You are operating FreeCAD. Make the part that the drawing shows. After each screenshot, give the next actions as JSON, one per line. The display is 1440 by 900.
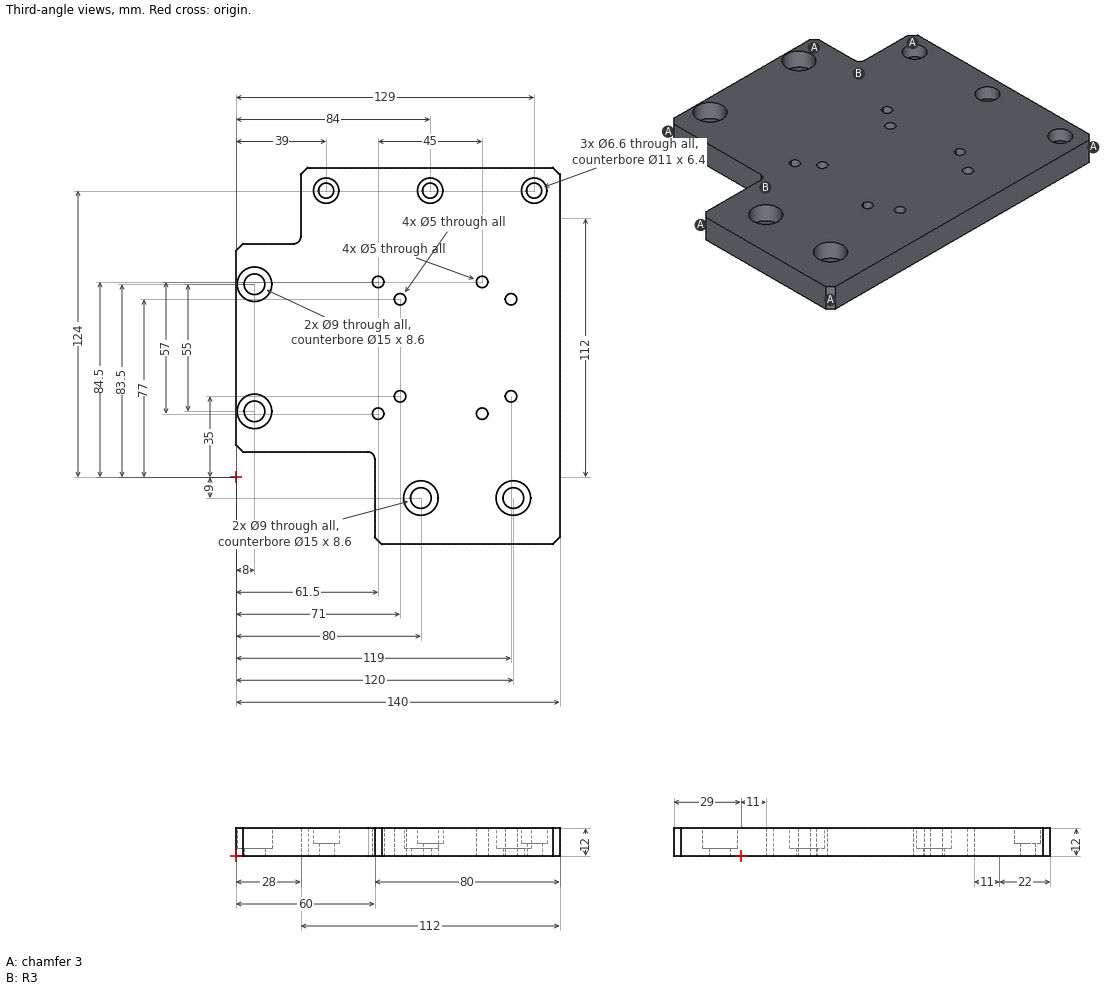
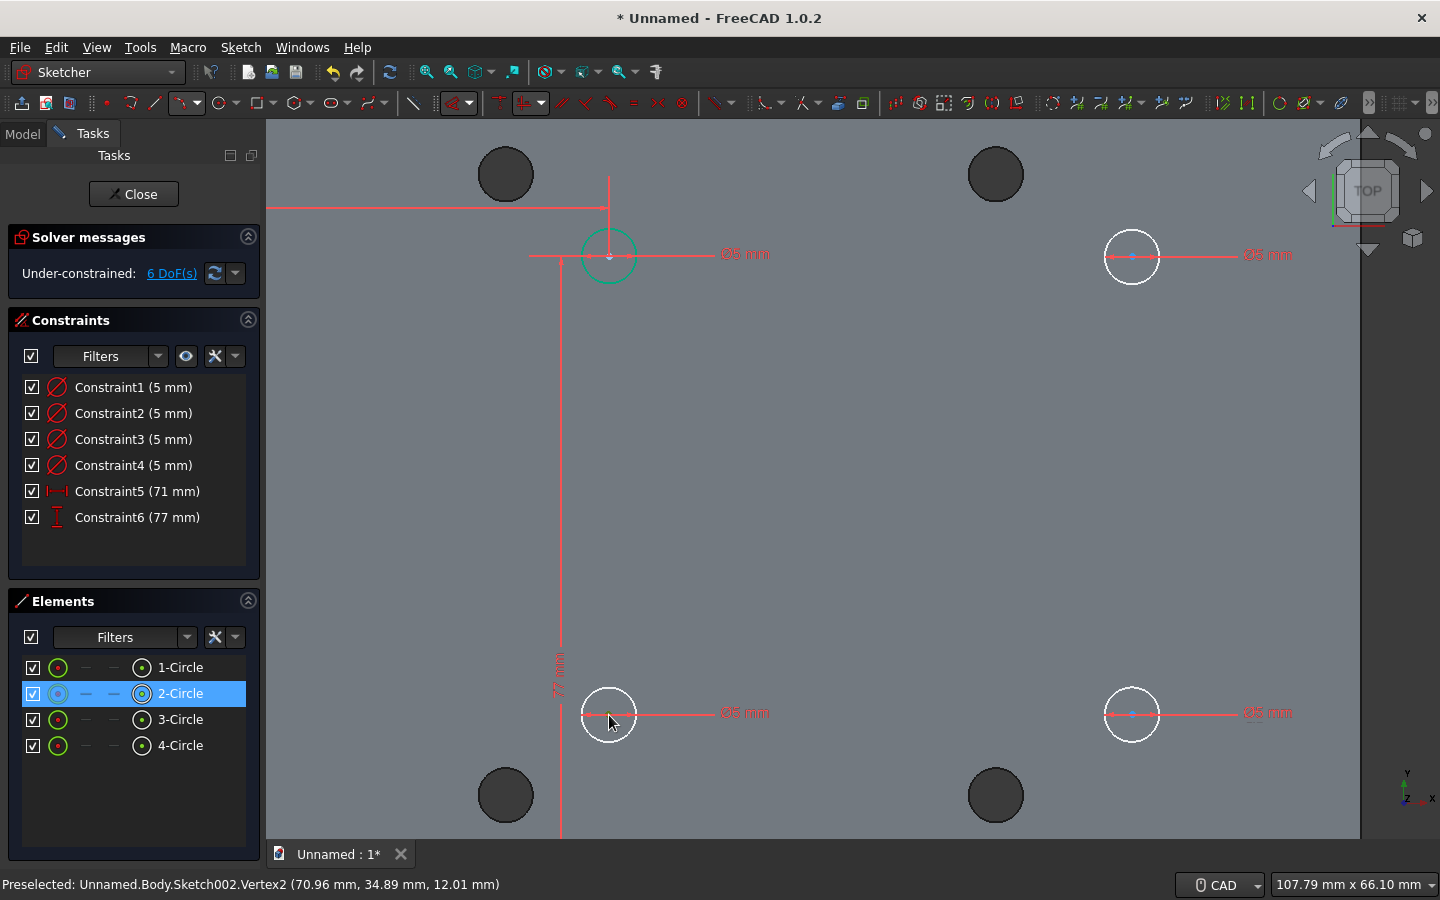
{"action": "left_click", "coordinate": [472, 104]}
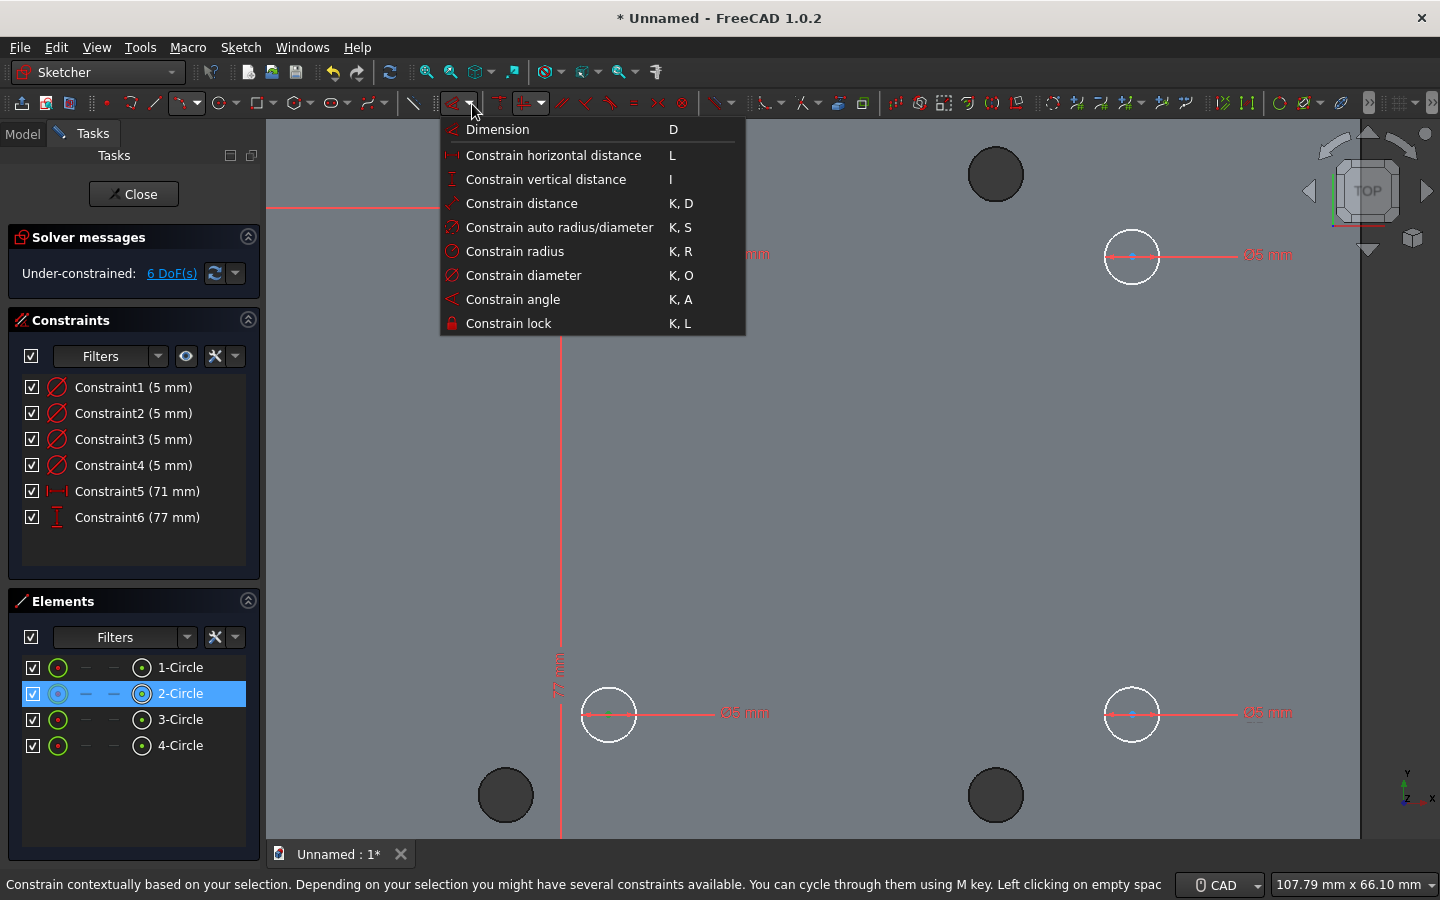
{"action": "left_click", "coordinate": [593, 155]}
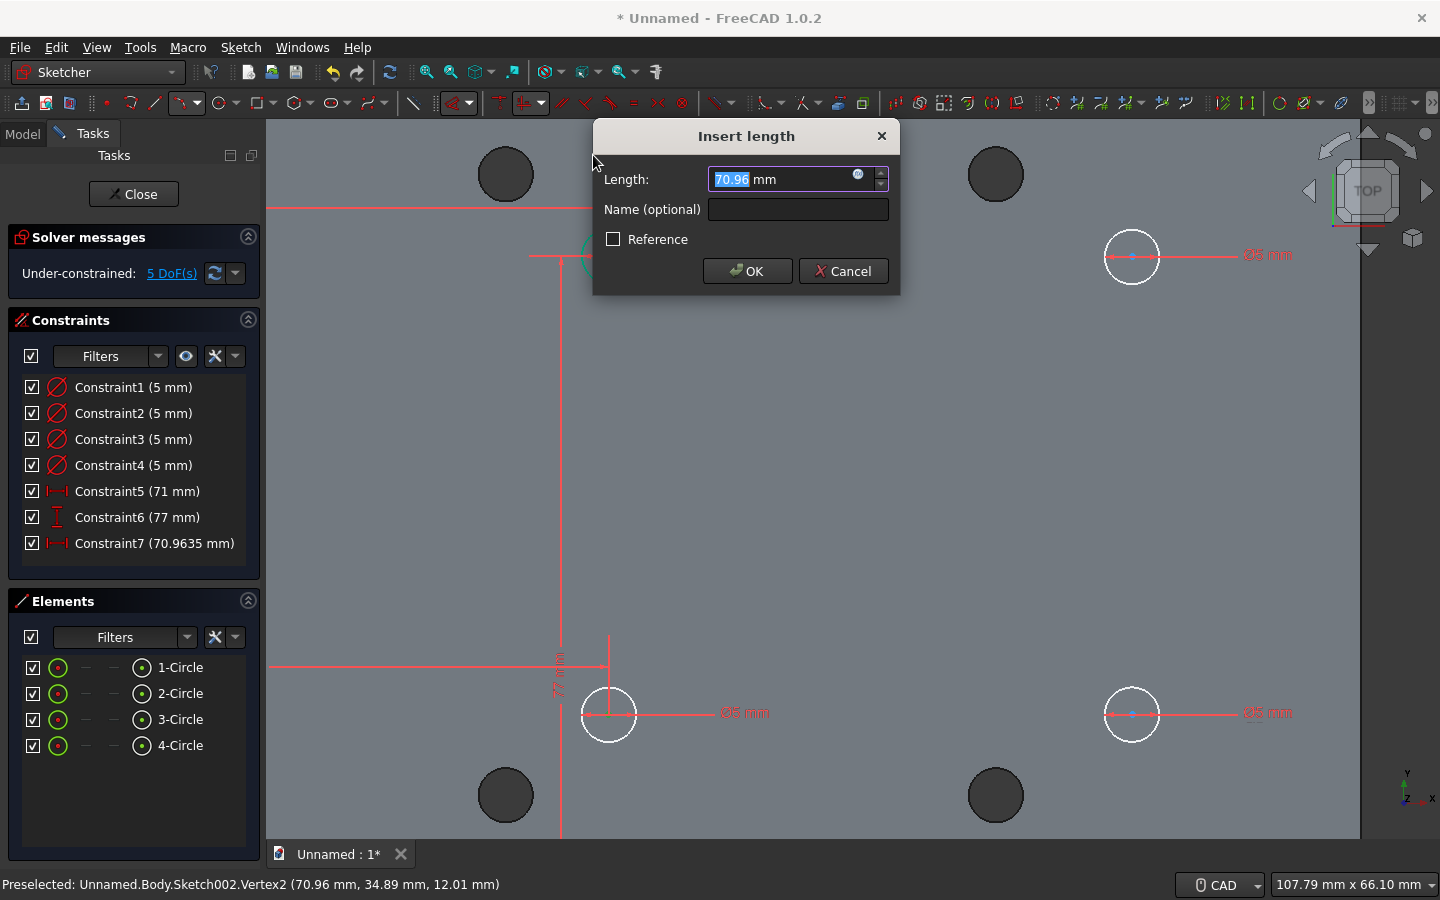
{"action": "type", "text": "71"}
{"action": "key", "text": "Return"}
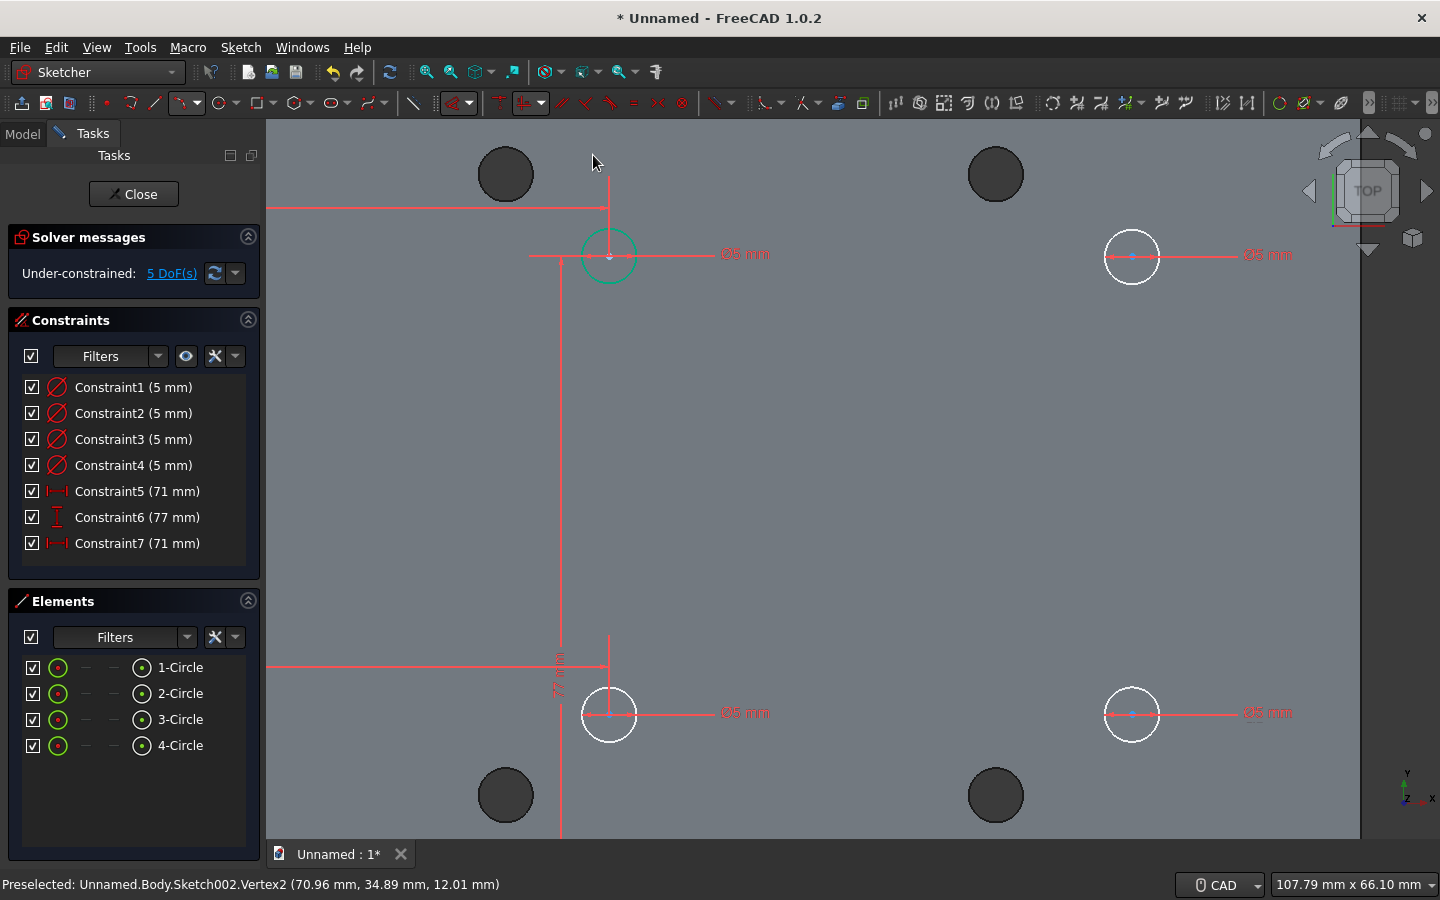
{"action": "left_click", "coordinate": [609, 715]}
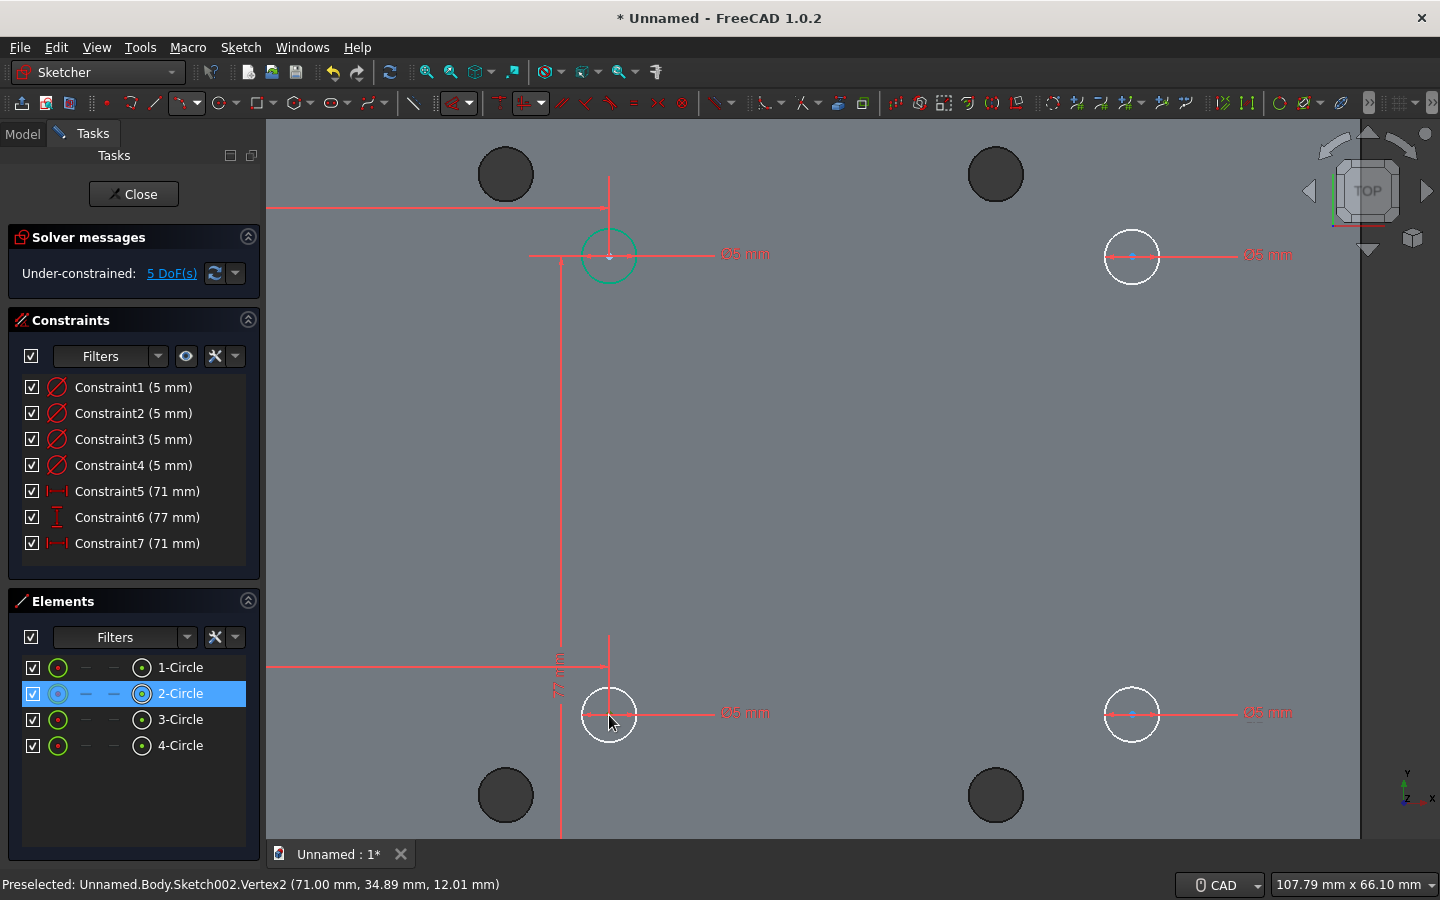
{"action": "left_click", "coordinate": [472, 104]}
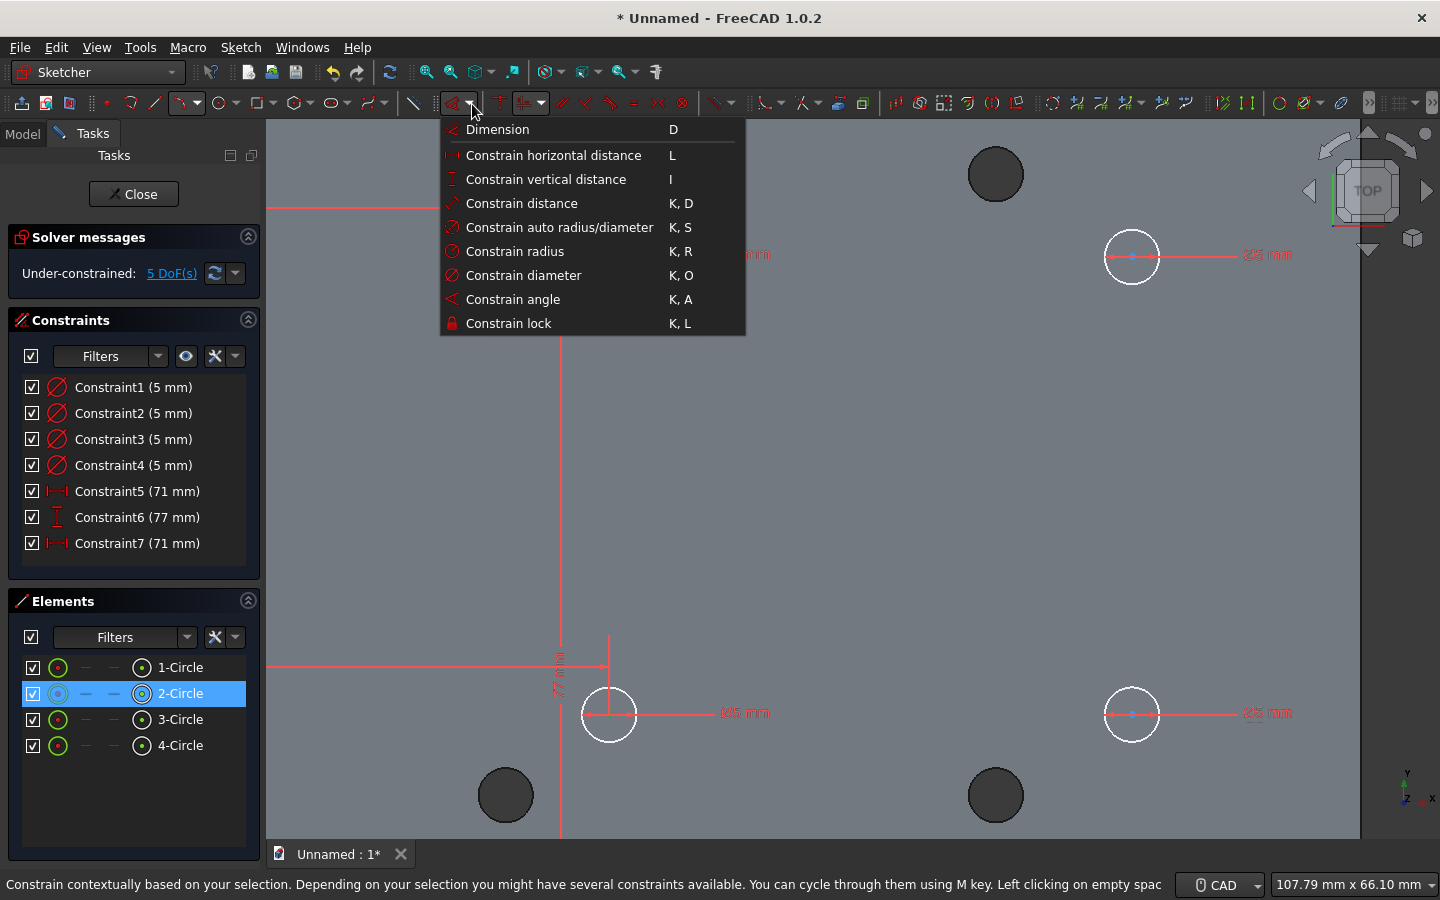
{"action": "left_click", "coordinate": [593, 179]}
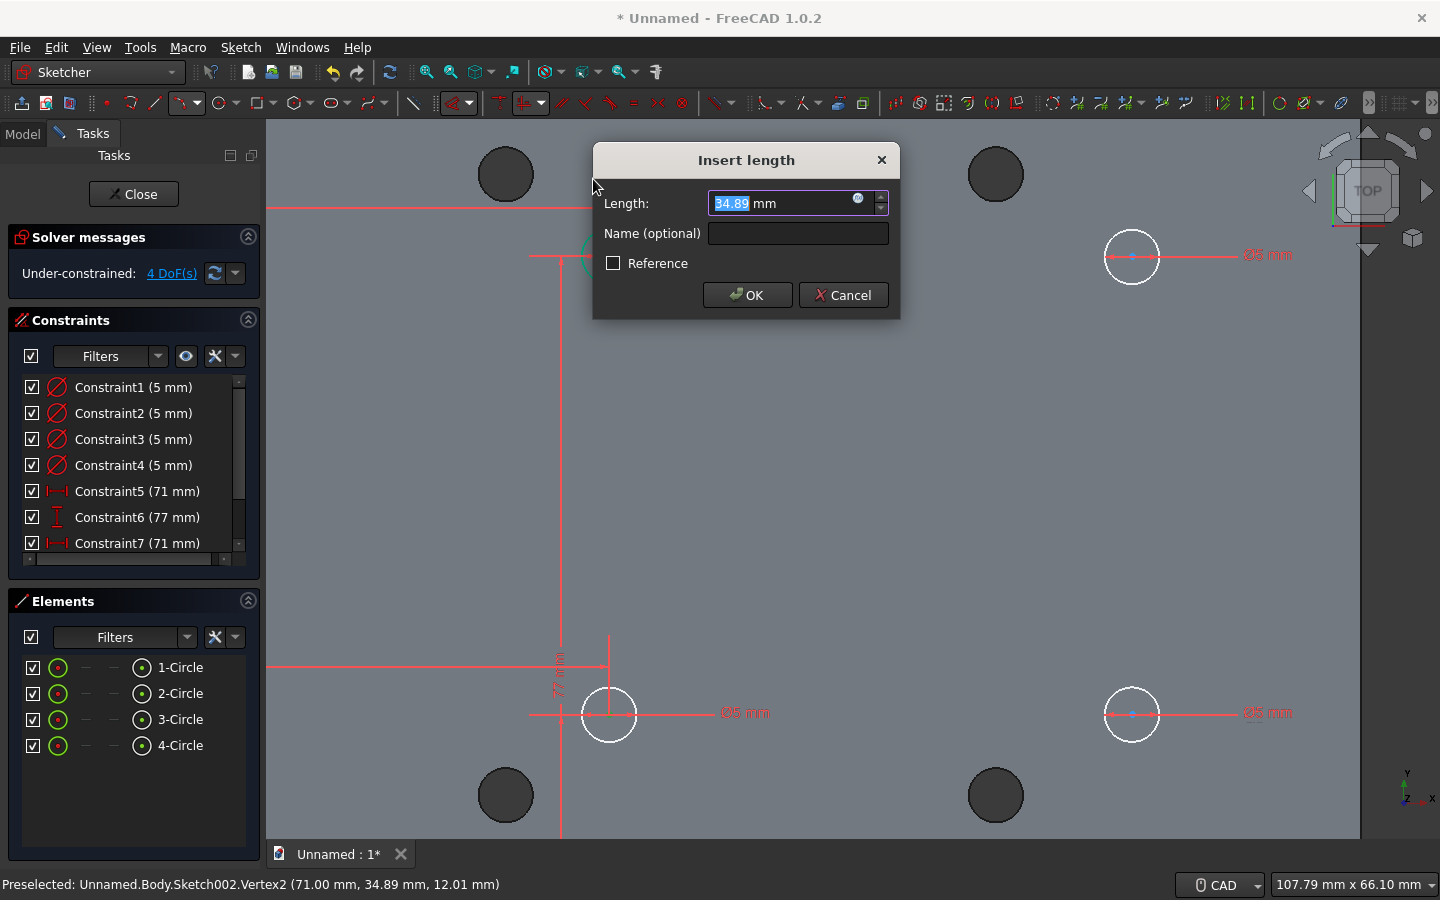
{"action": "type", "text": "35"}
{"action": "key", "text": "Return"}